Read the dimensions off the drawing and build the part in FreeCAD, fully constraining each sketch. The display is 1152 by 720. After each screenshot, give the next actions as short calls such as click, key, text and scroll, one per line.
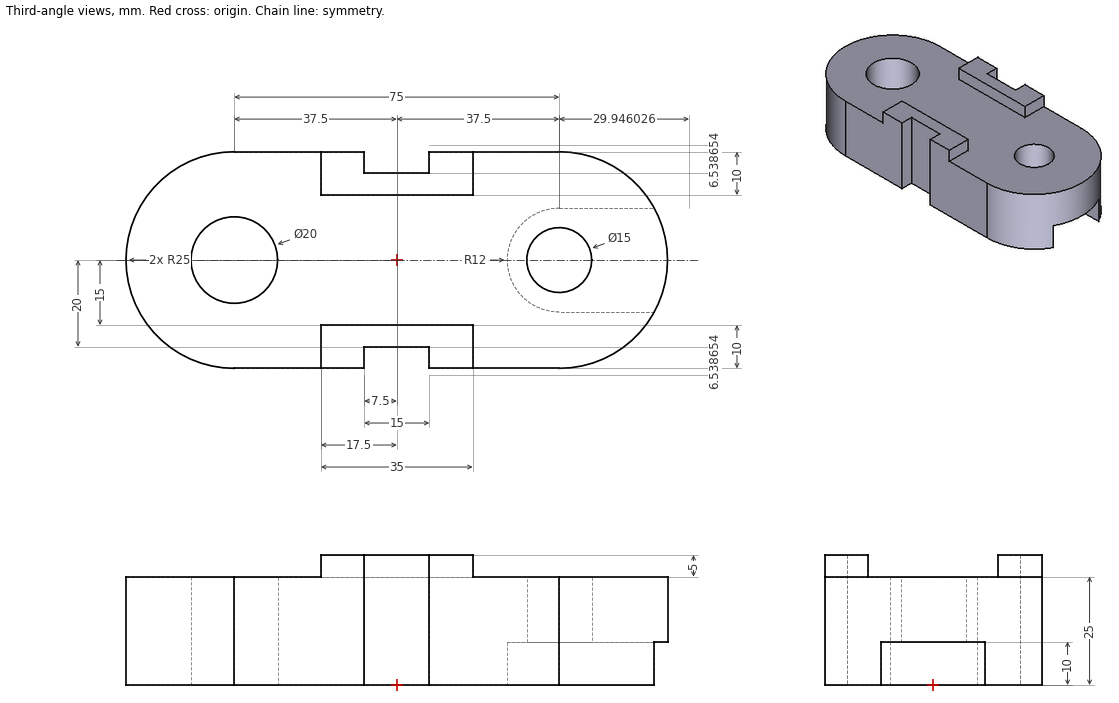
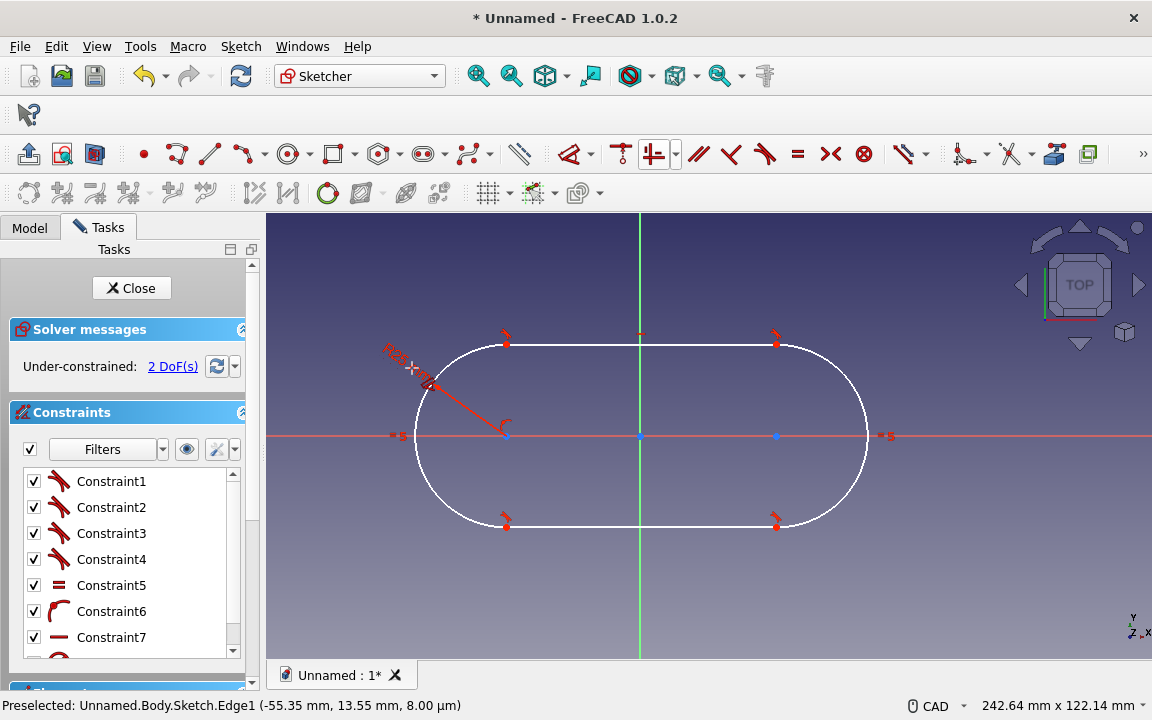
click(587, 345)
click(579, 311)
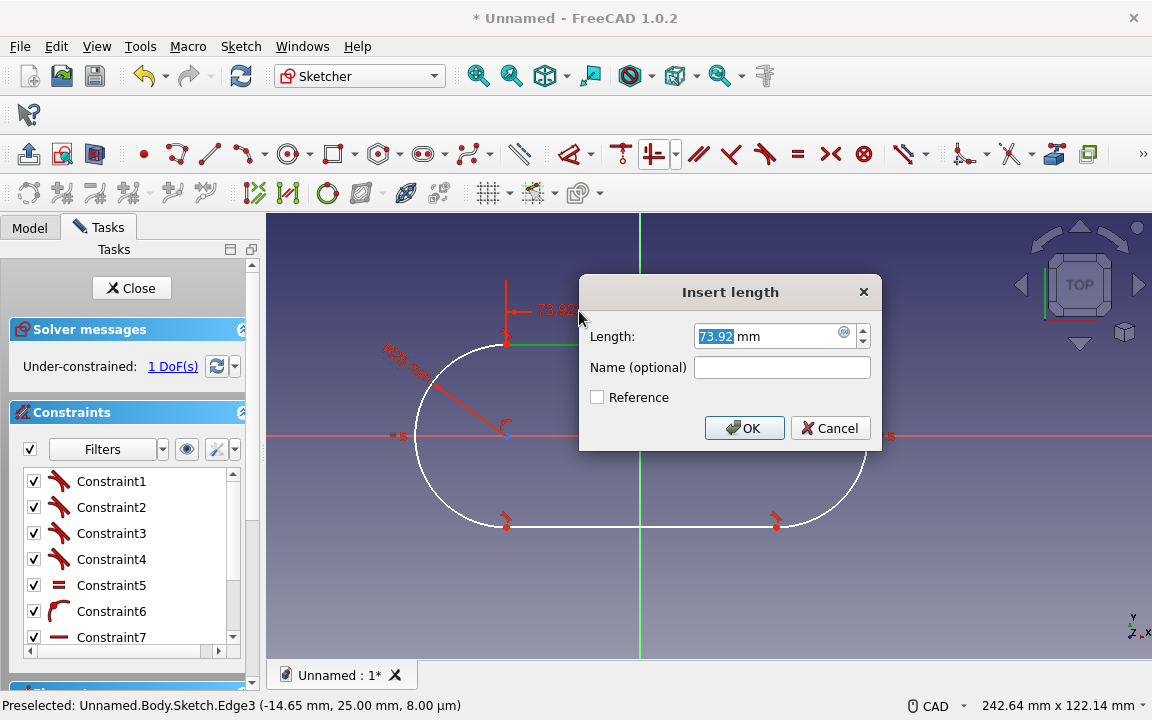
text(75)
key(Return)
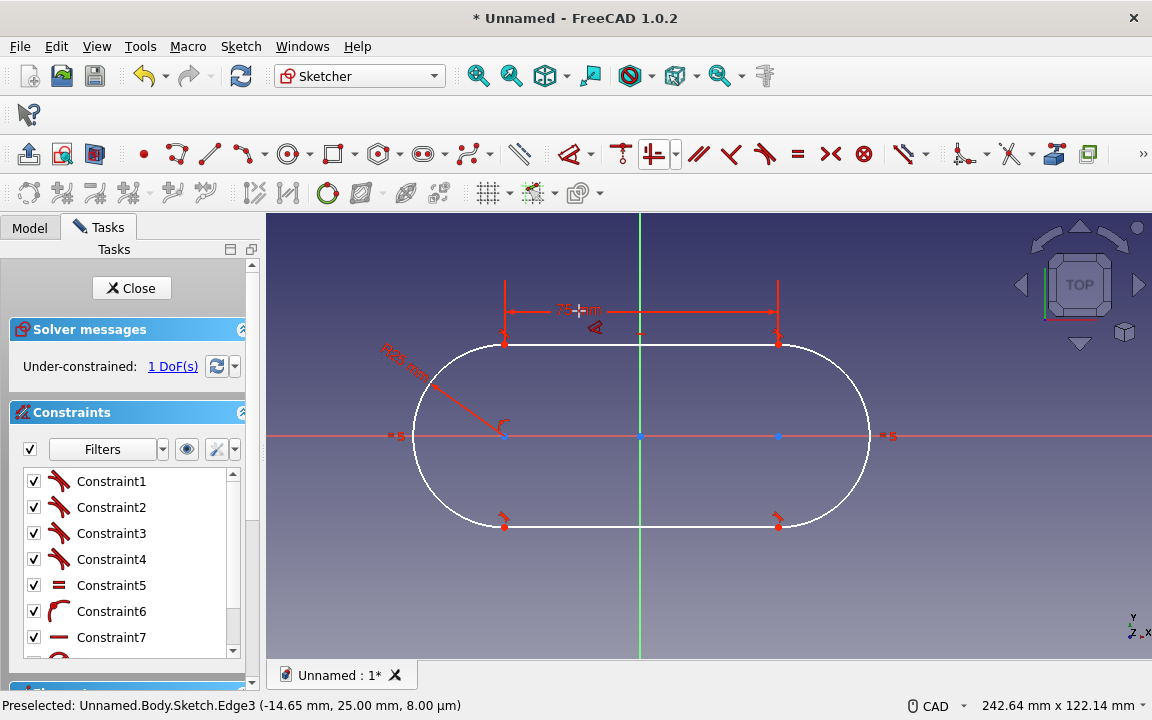
click(505, 345)
click(573, 470)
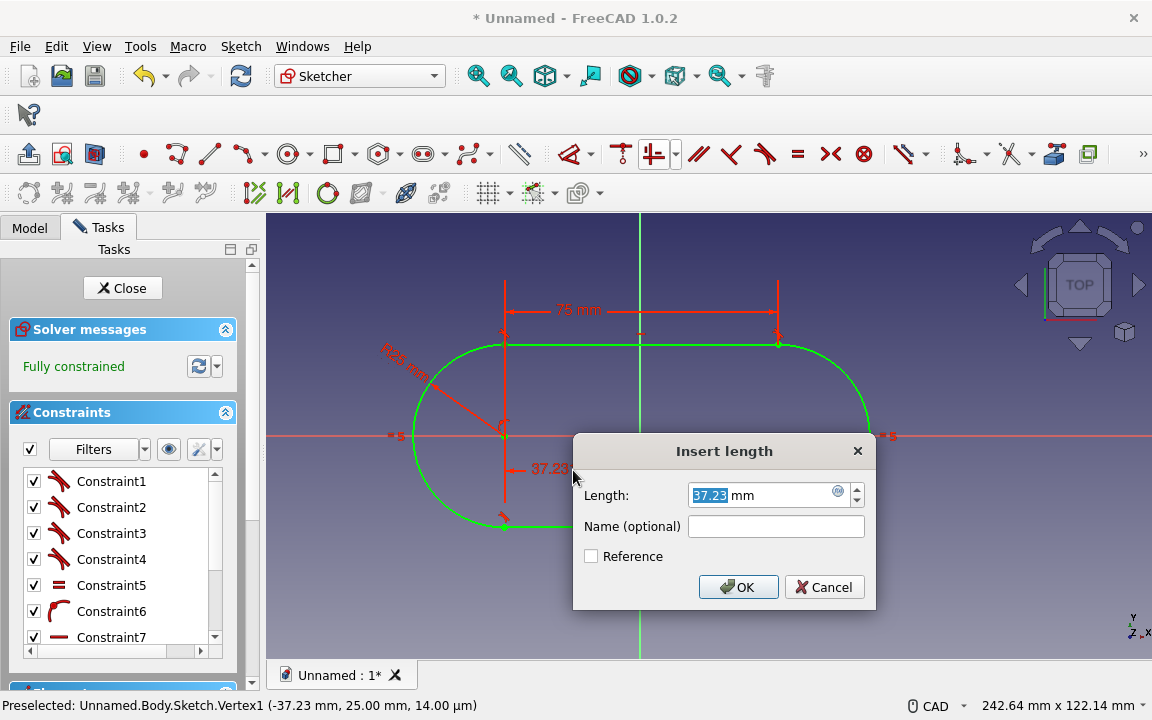
text(37.5)
key(Return)
key(Escape)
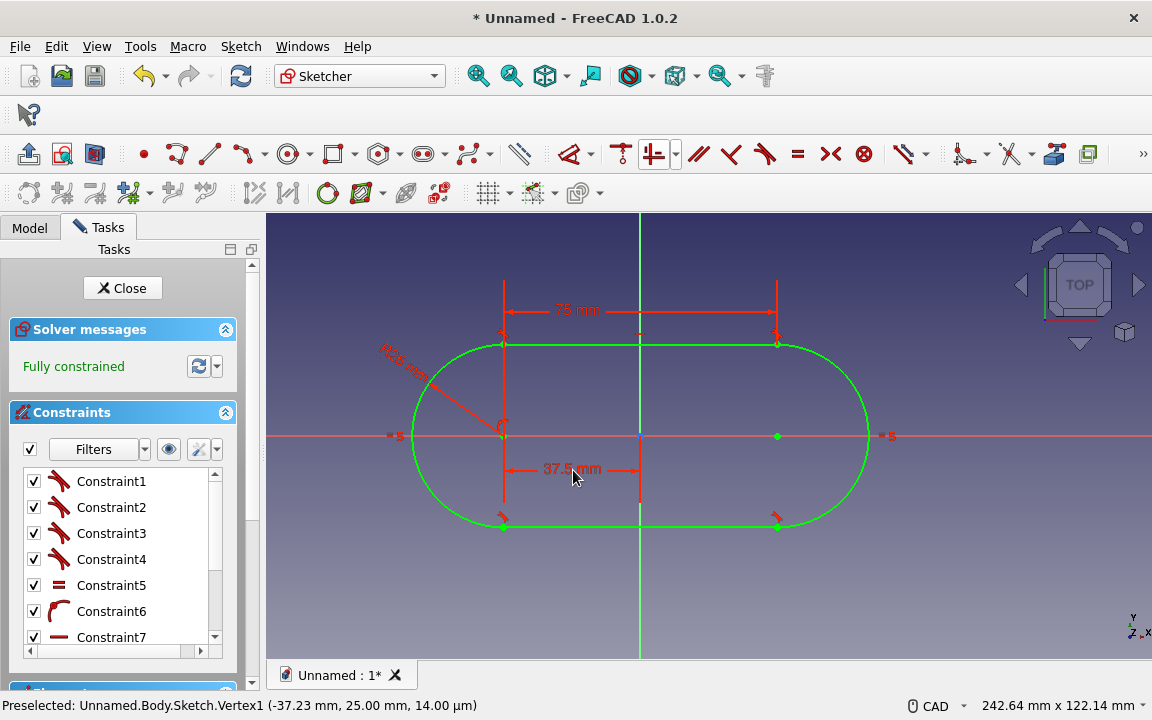
click(123, 288)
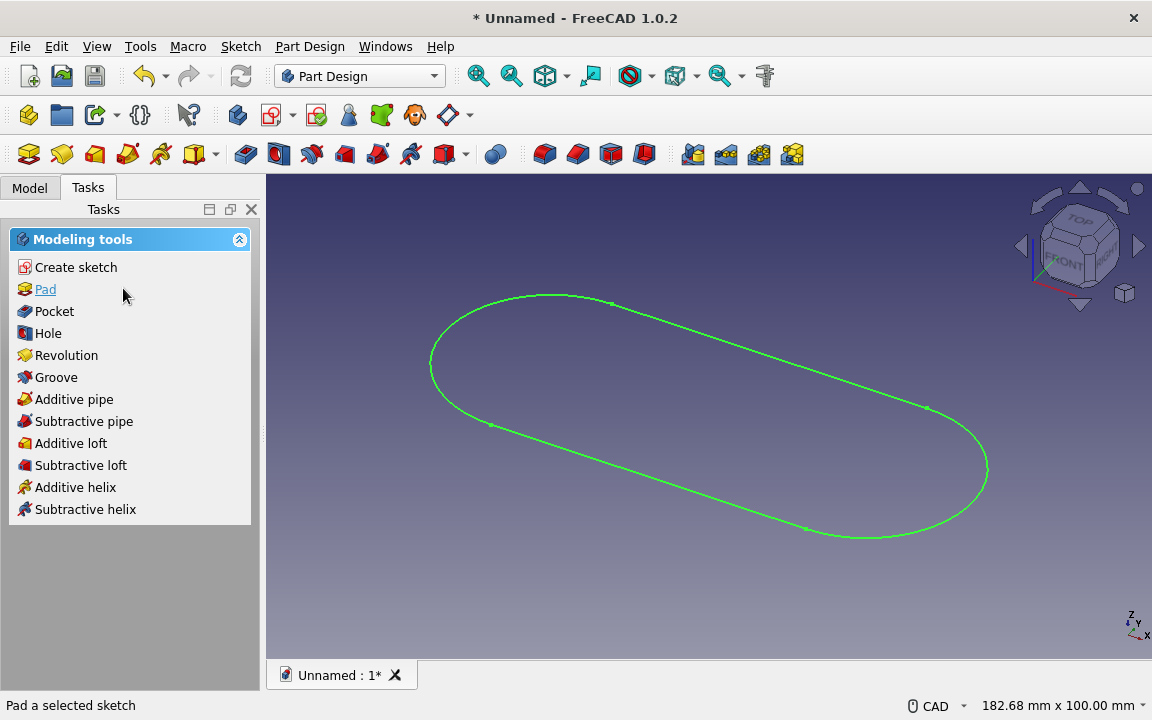
click(29, 154)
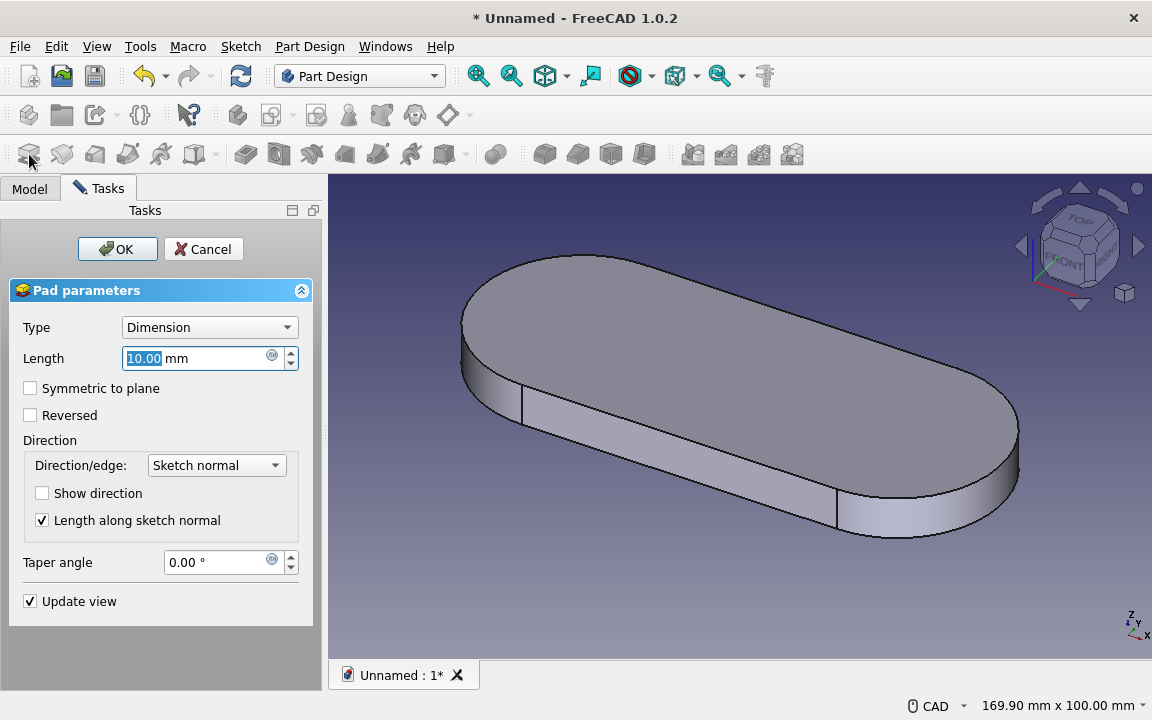
text(25)
key(Tab)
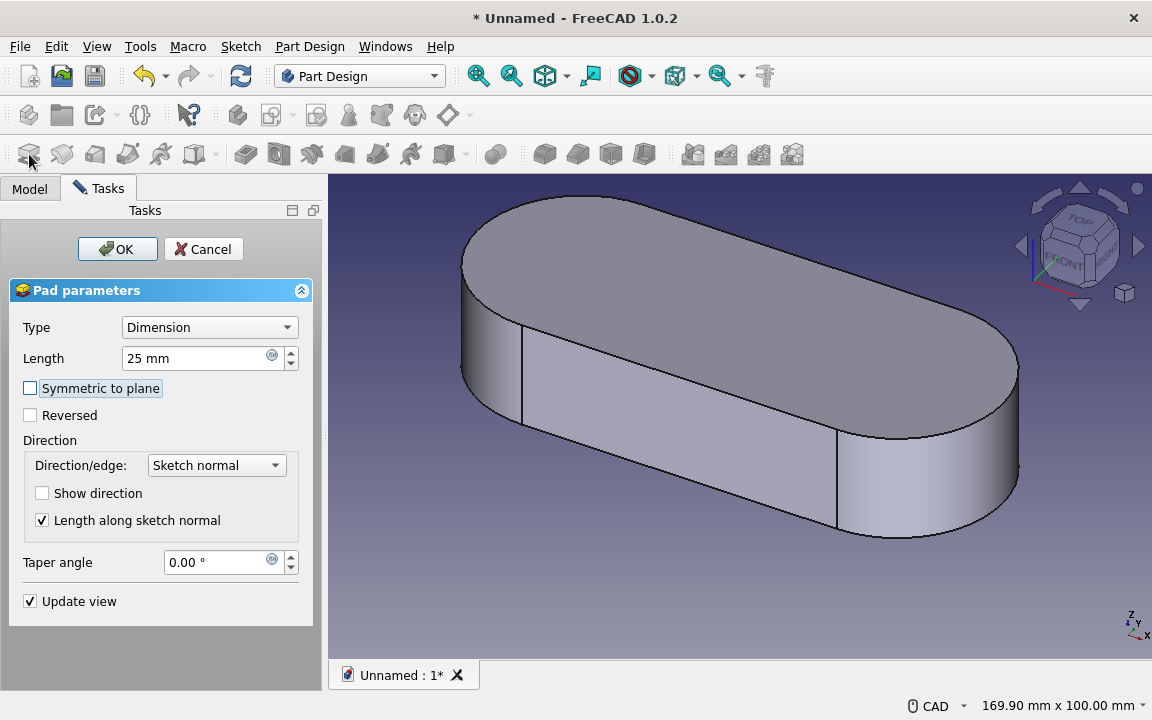
click(118, 249)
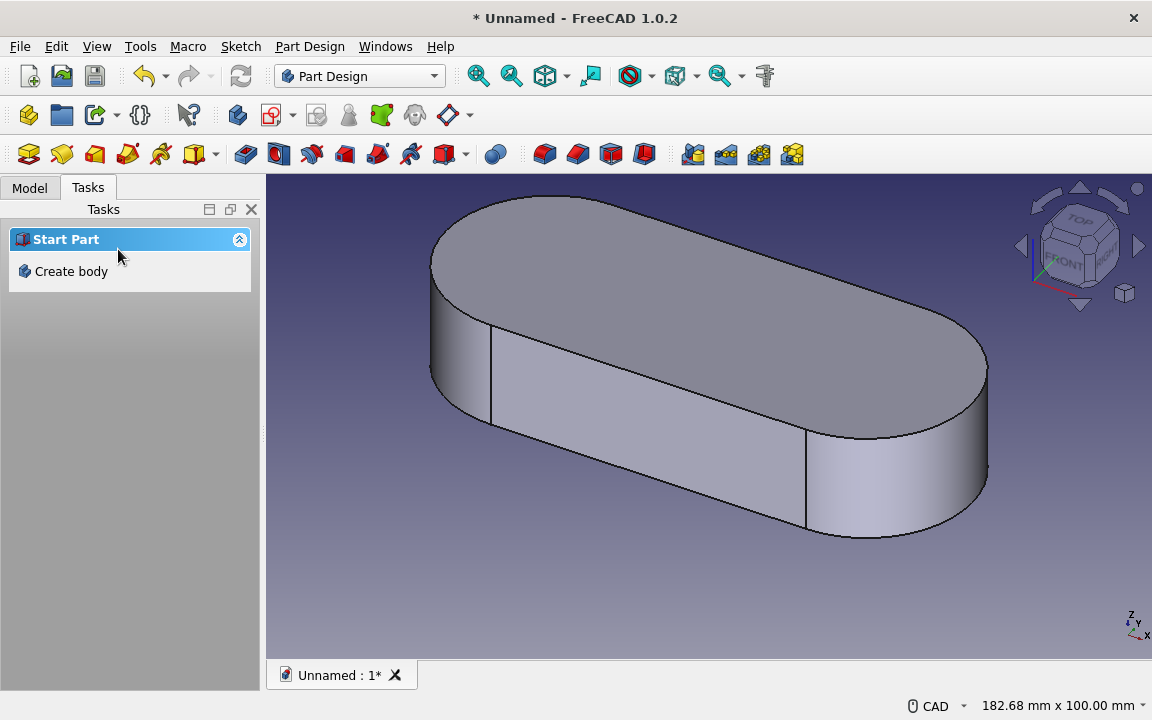
key(v)
key(f)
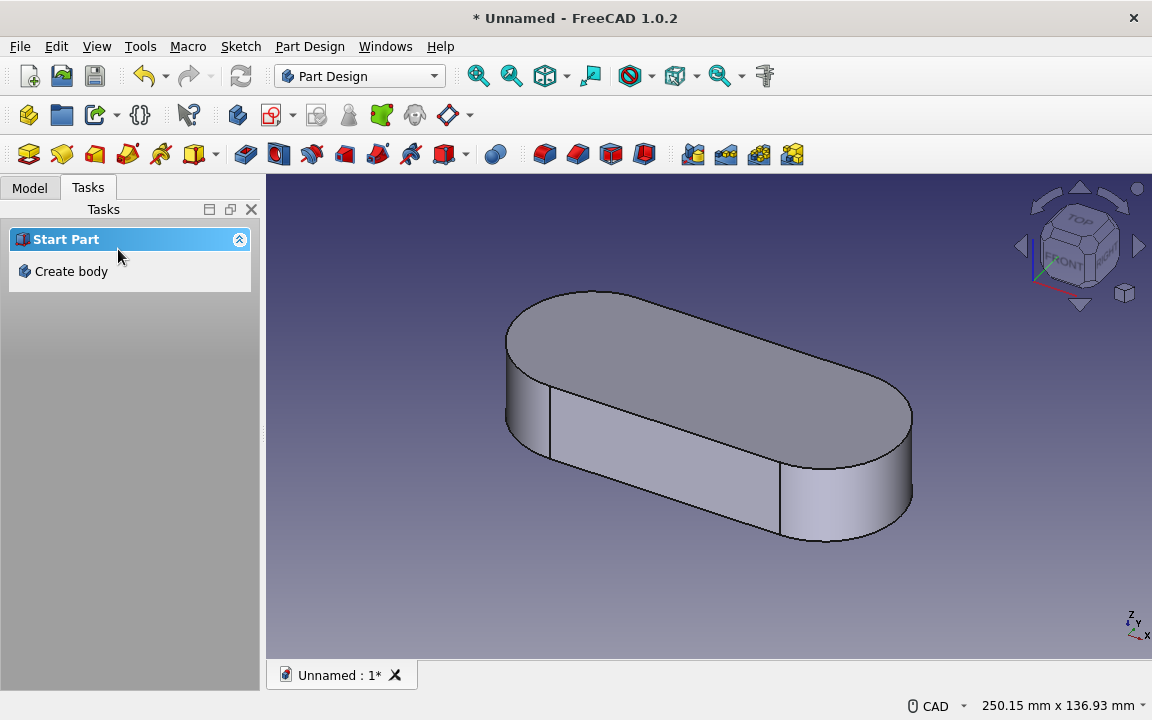
click(819, 416)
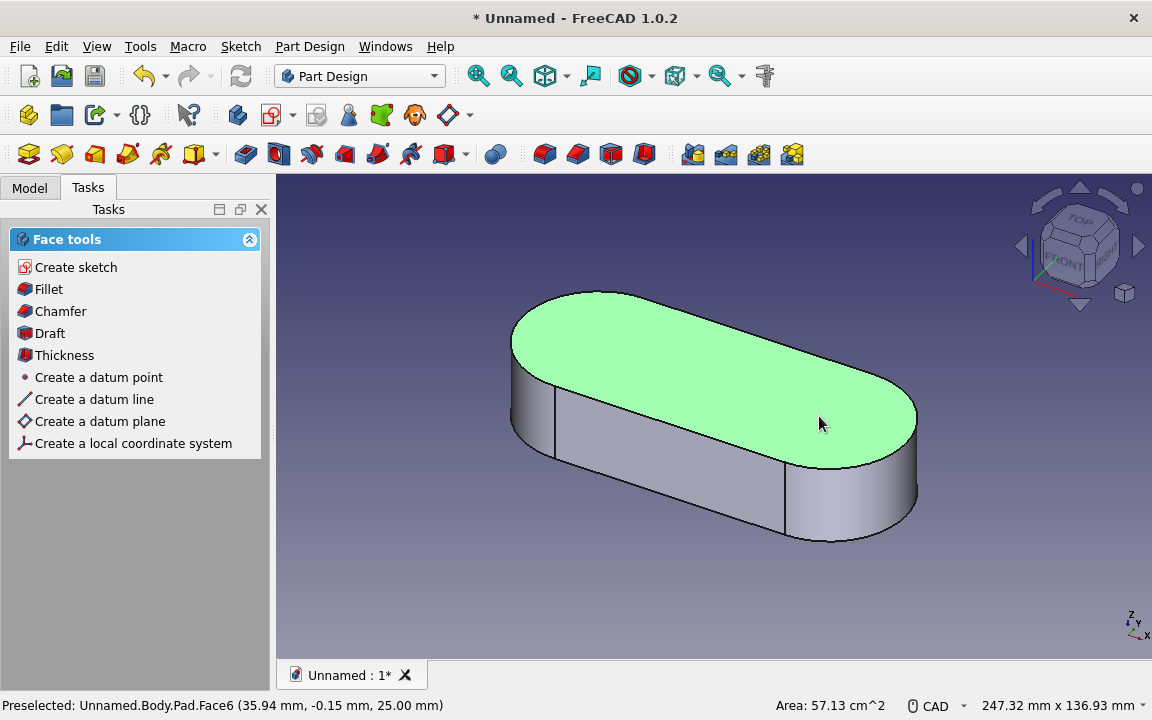
click(270, 116)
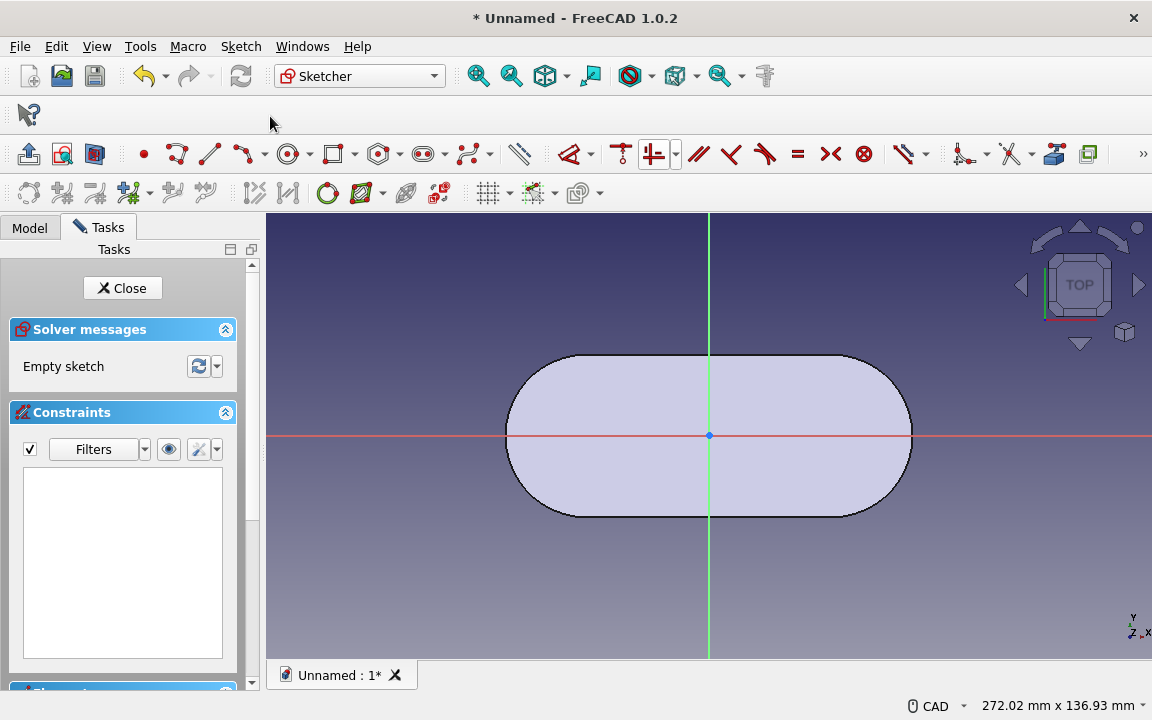
scroll(792, 436, up, 3)